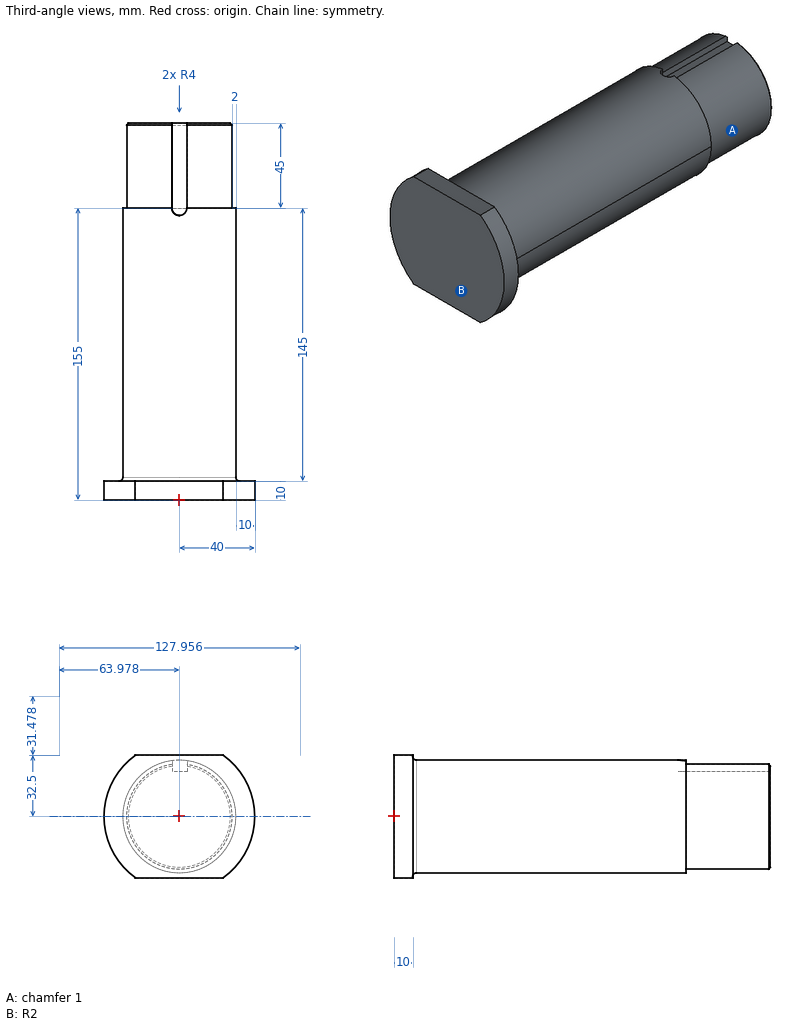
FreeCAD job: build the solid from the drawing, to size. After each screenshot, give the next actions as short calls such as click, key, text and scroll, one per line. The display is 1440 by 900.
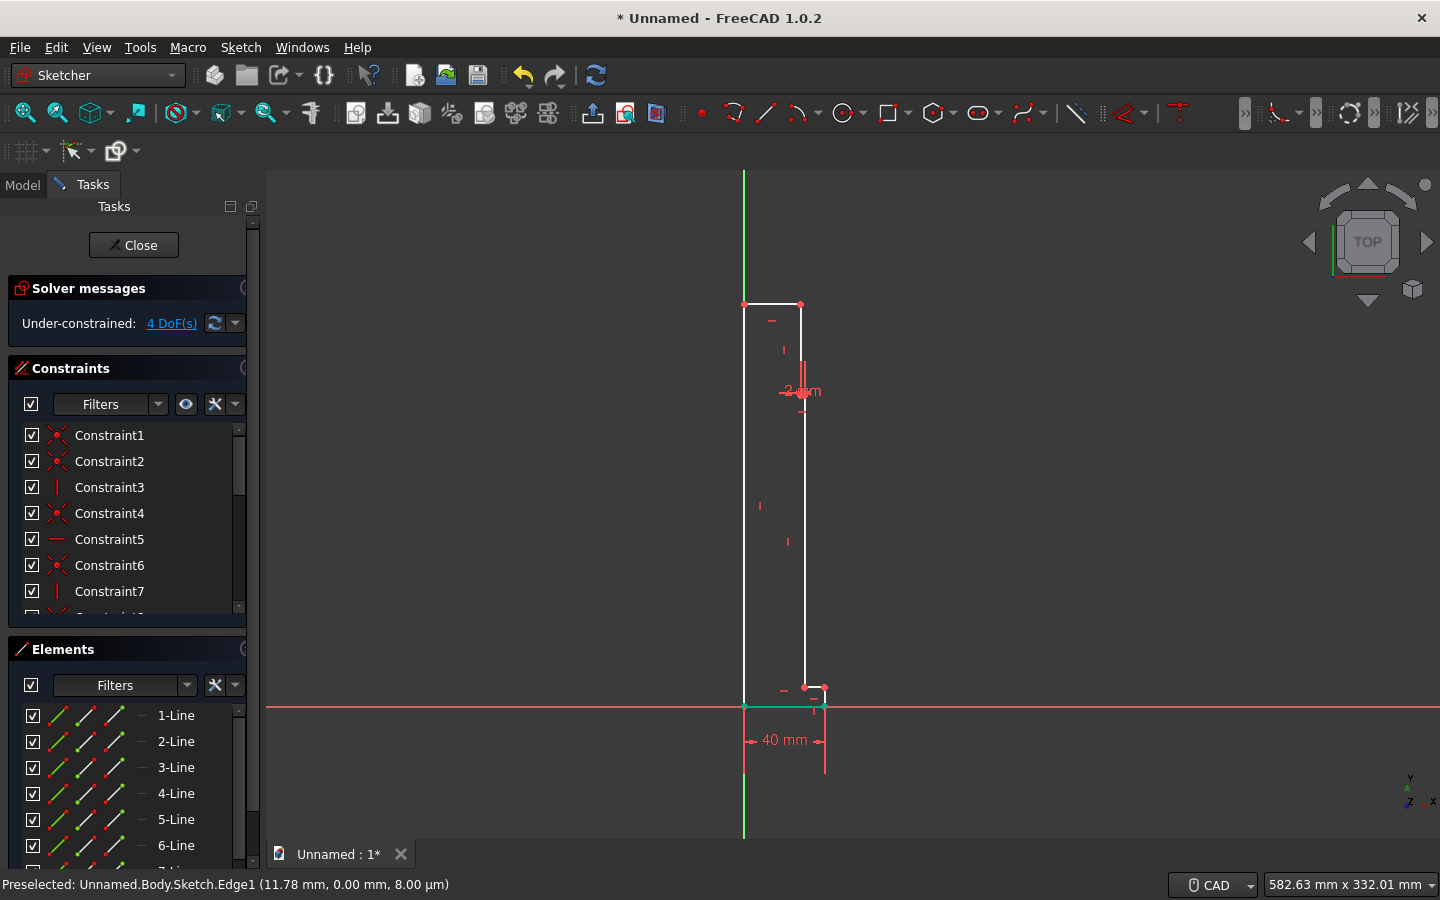
scroll(825, 697, up, 4)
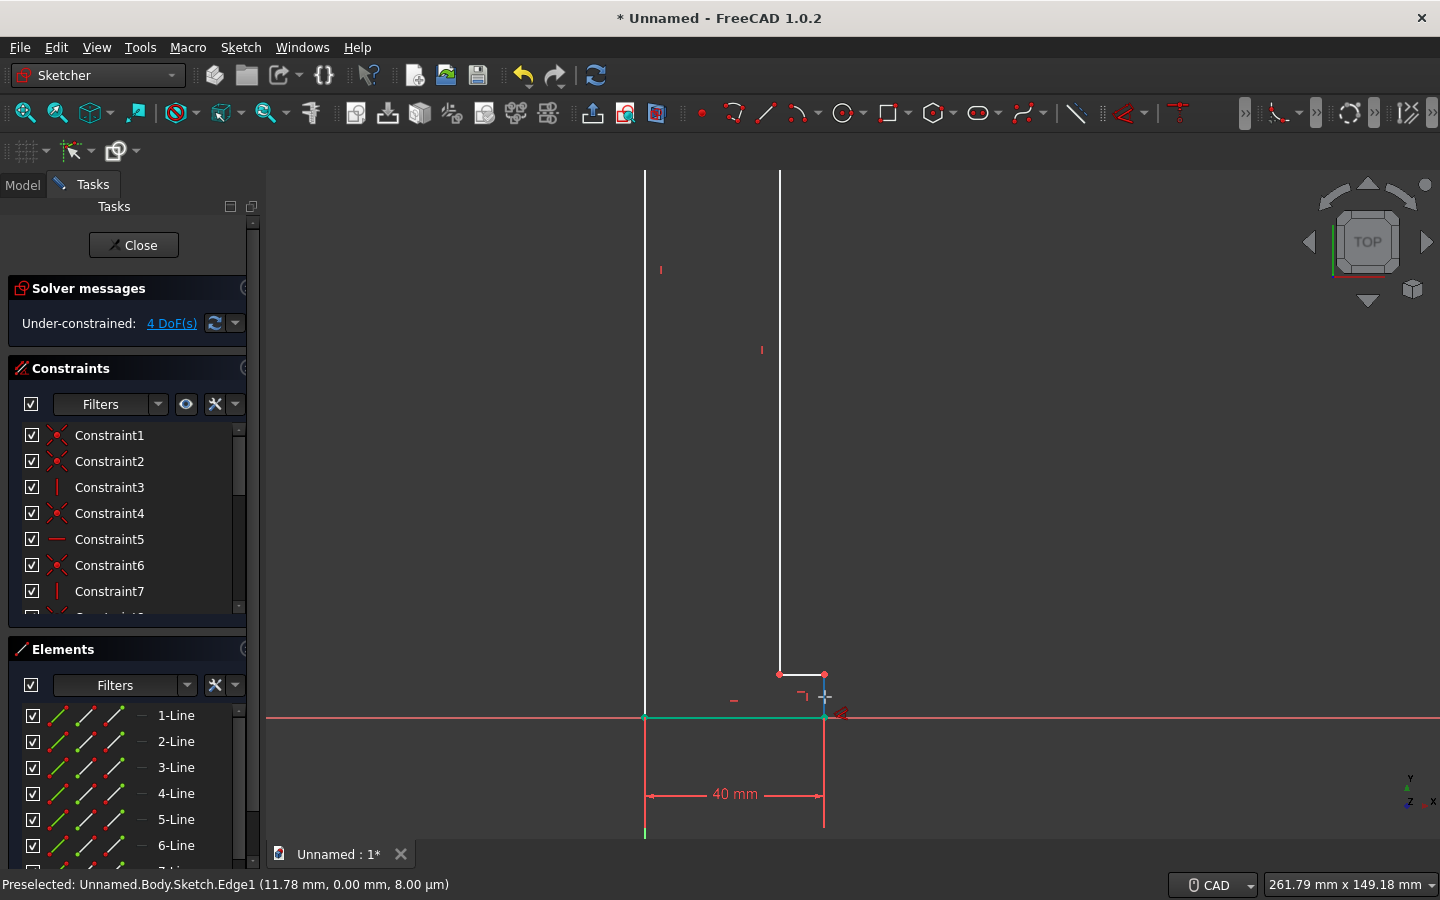
click(824, 696)
click(858, 696)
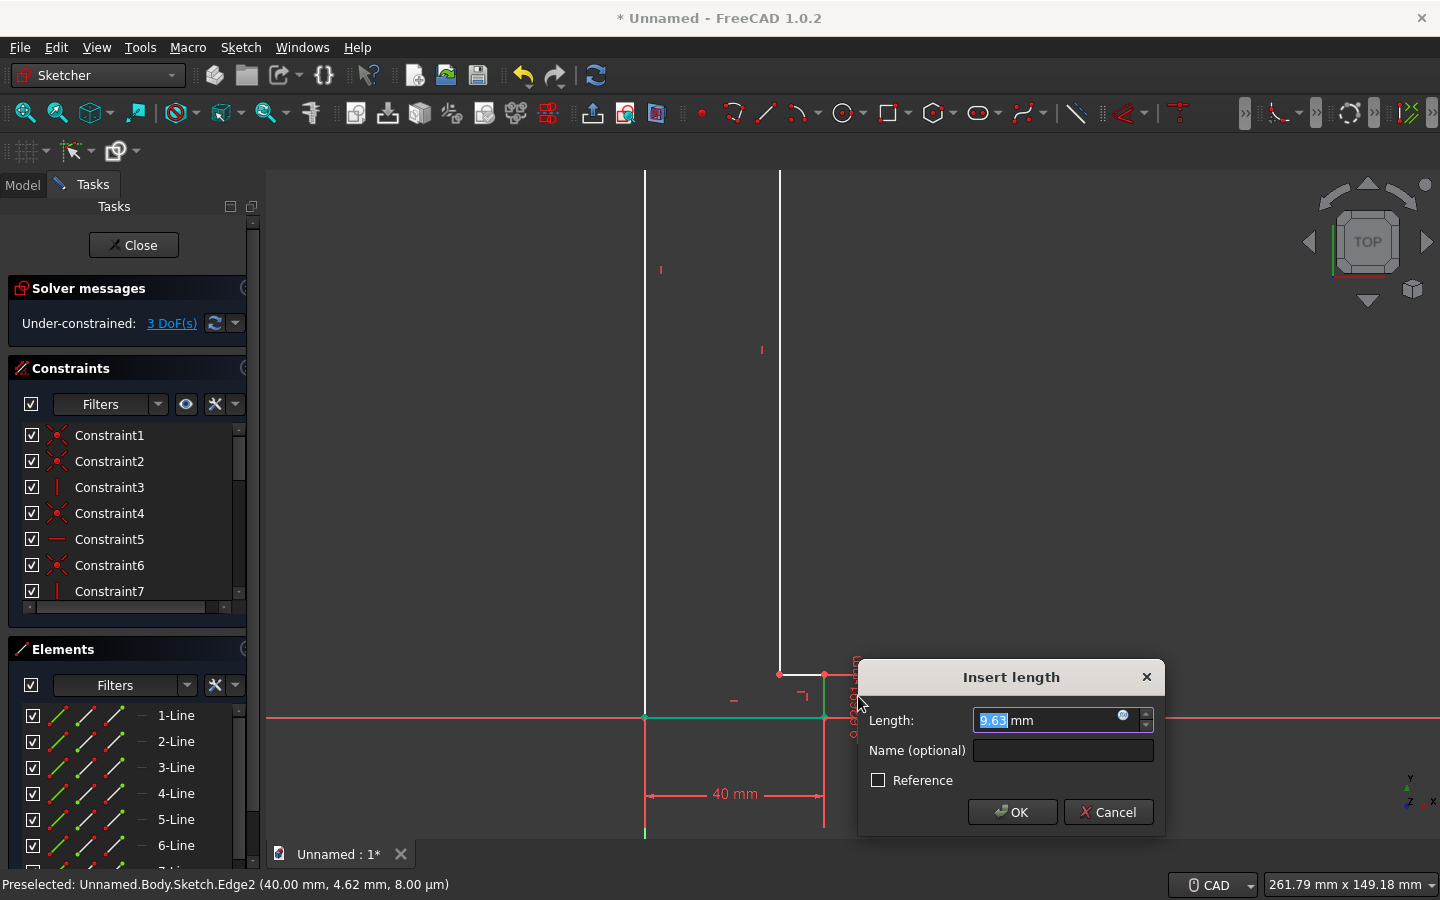
text(10)
key(Return)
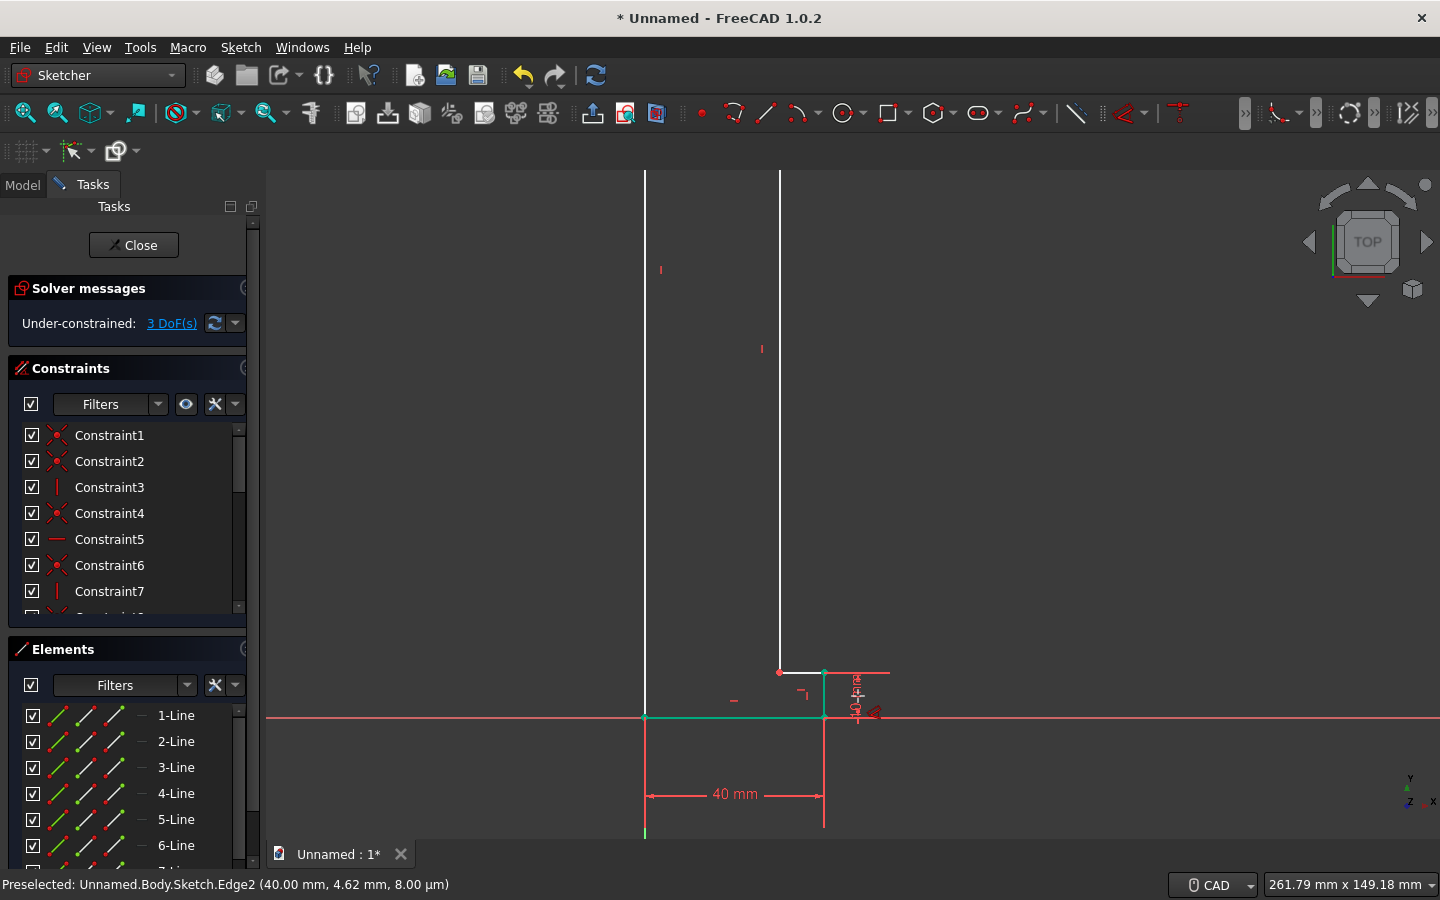
click(811, 673)
click(802, 639)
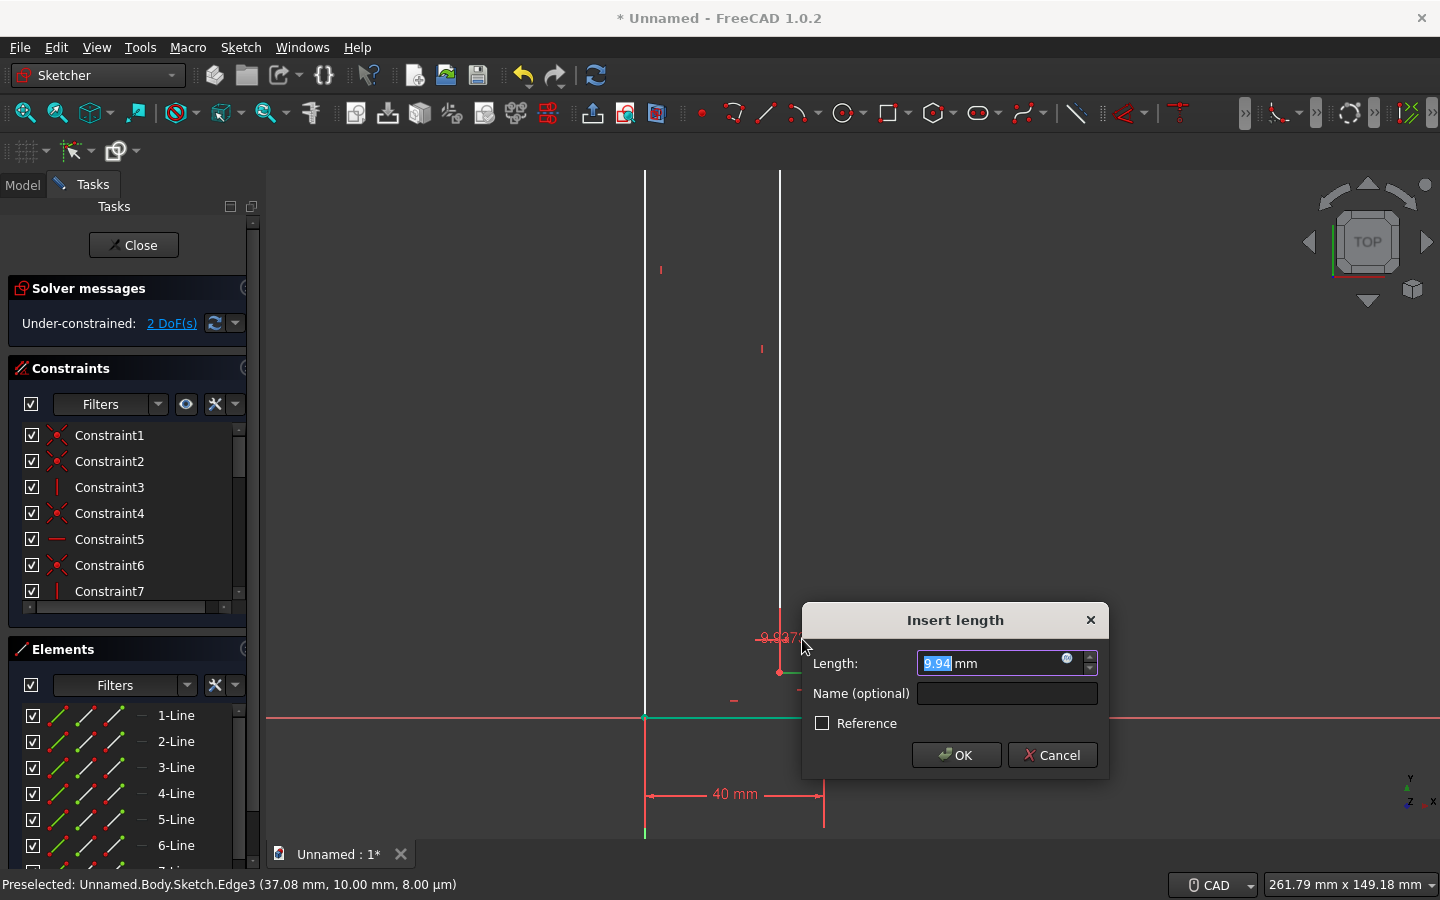
text(10)
key(Return)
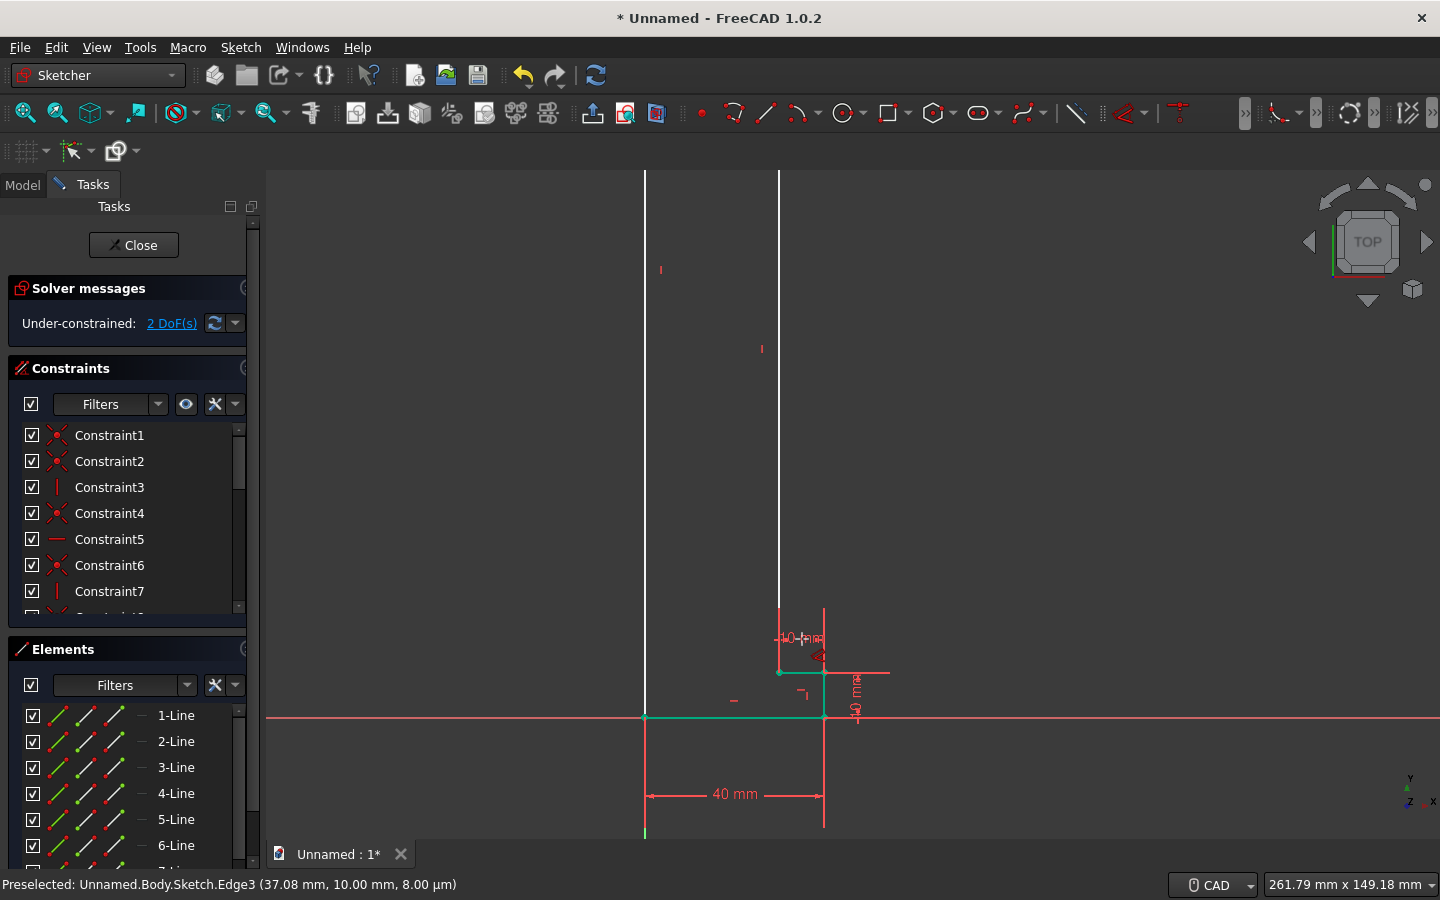
scroll(825, 696, down, 4)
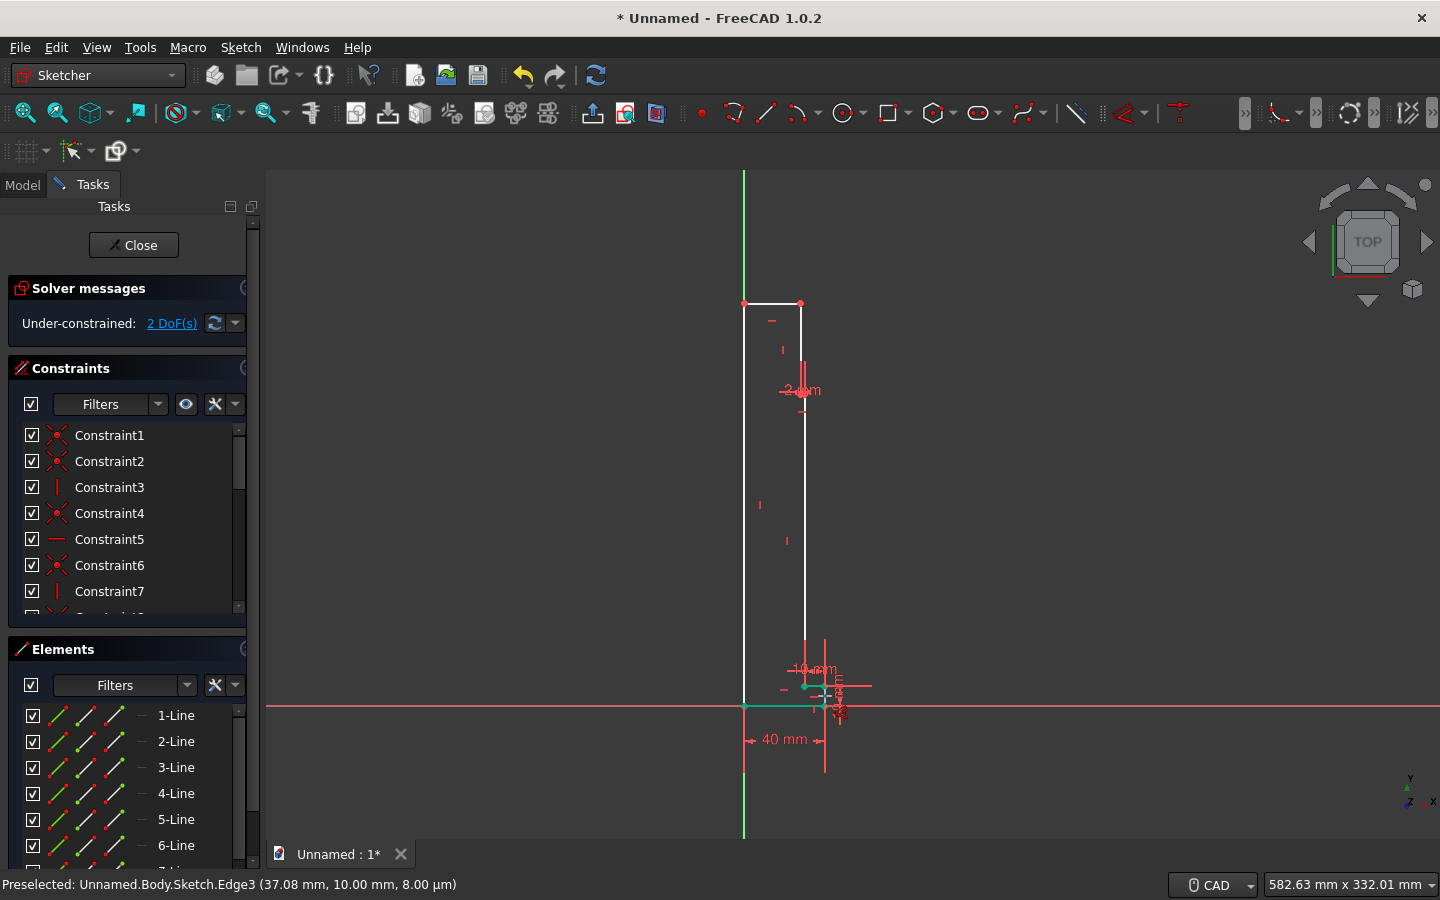
click(801, 367)
click(835, 349)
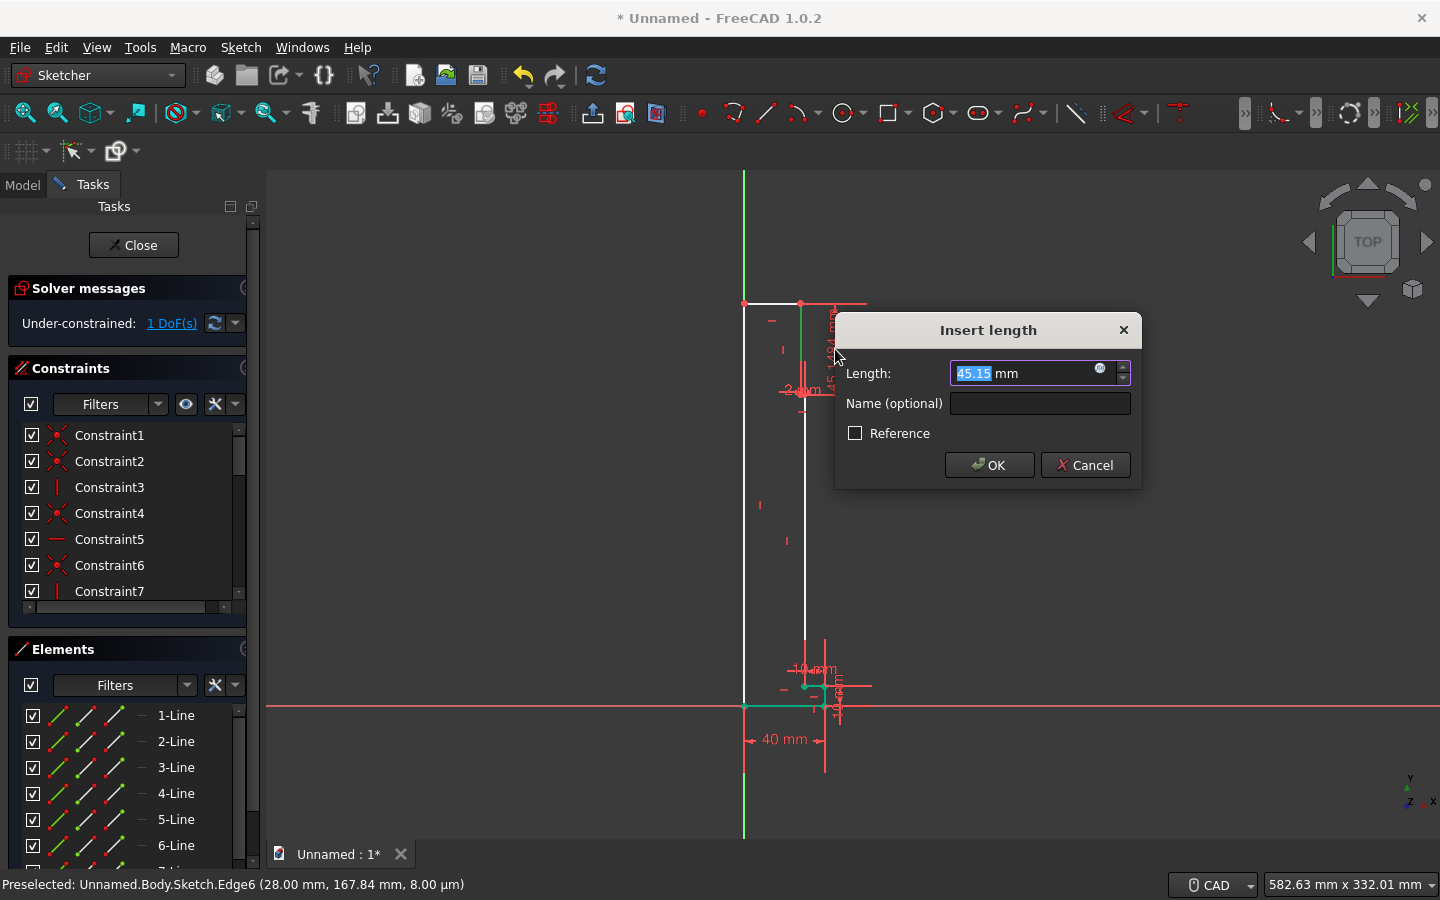
text(45)
key(Return)